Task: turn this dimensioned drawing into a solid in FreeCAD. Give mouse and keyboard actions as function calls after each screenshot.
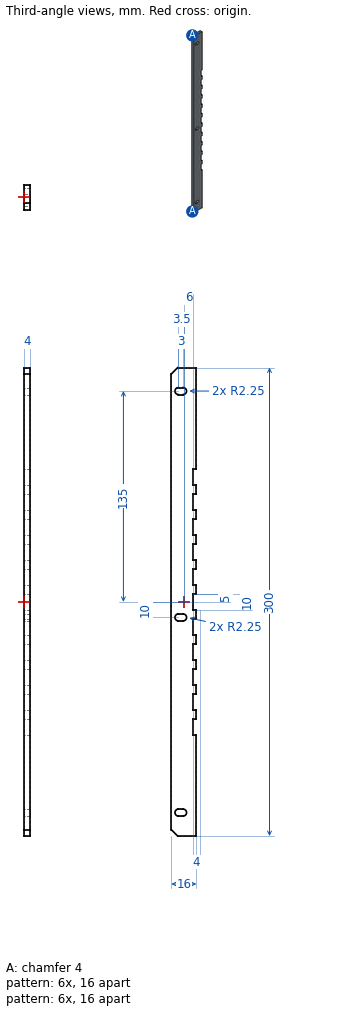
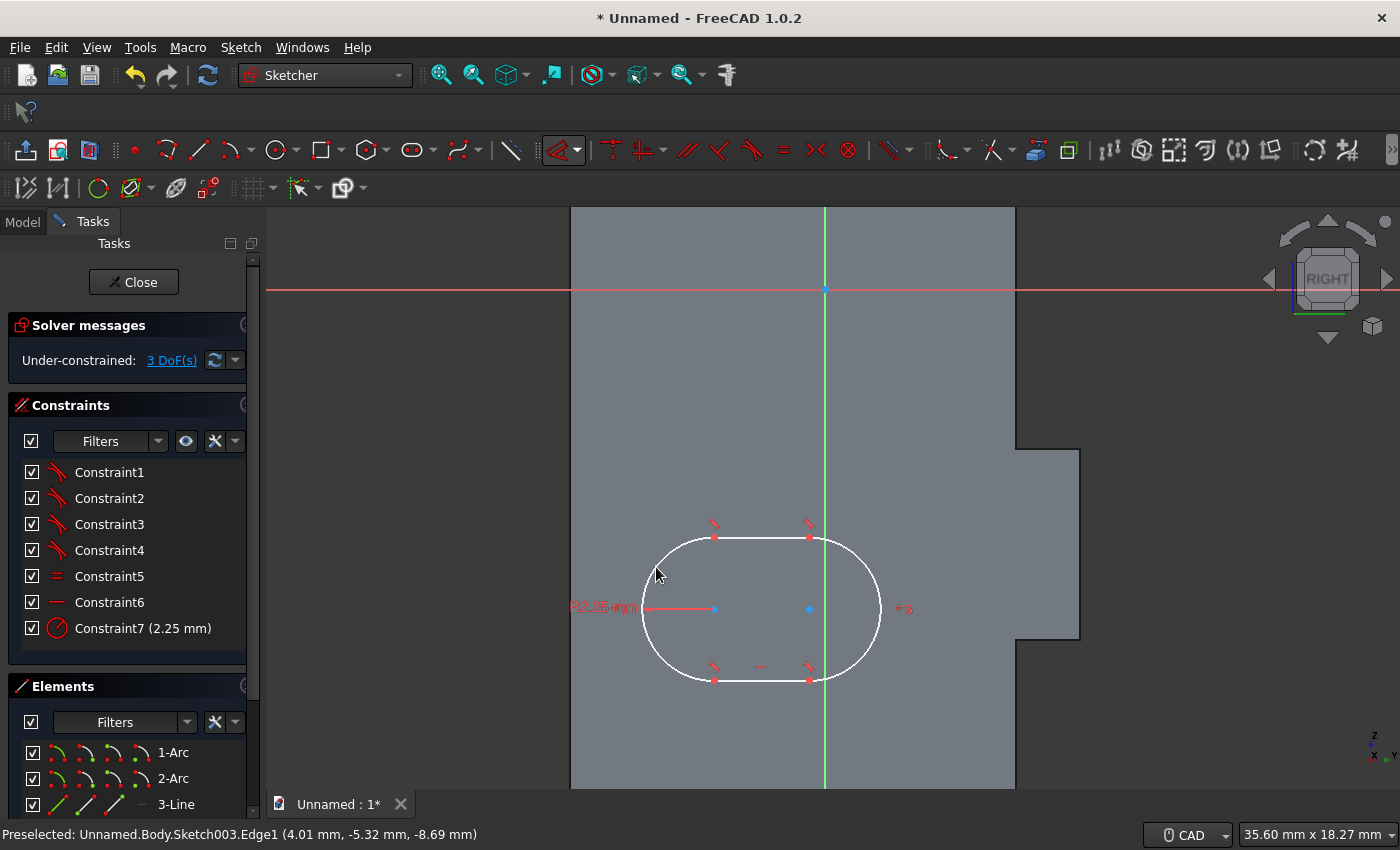
click(743, 538)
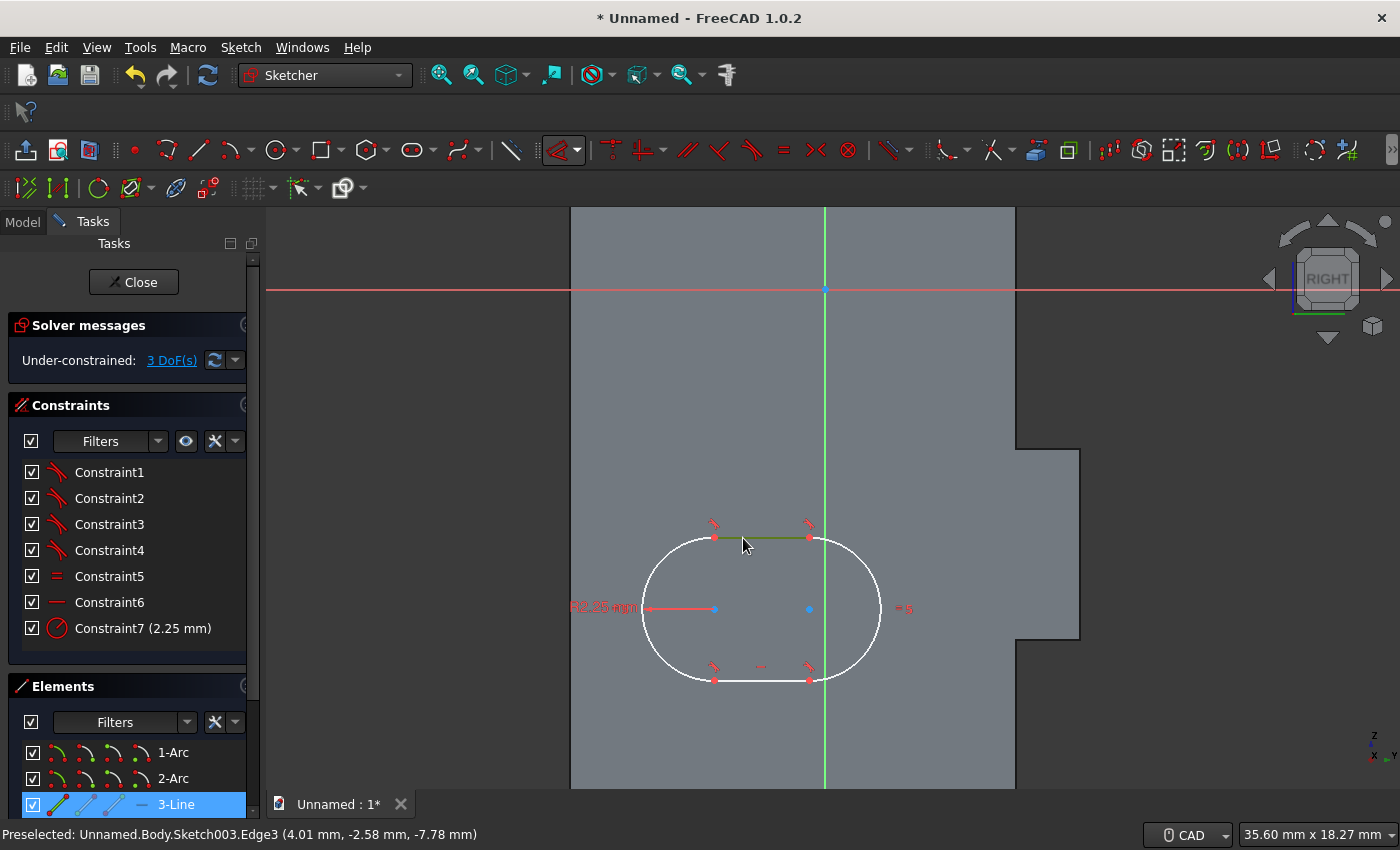
key(l)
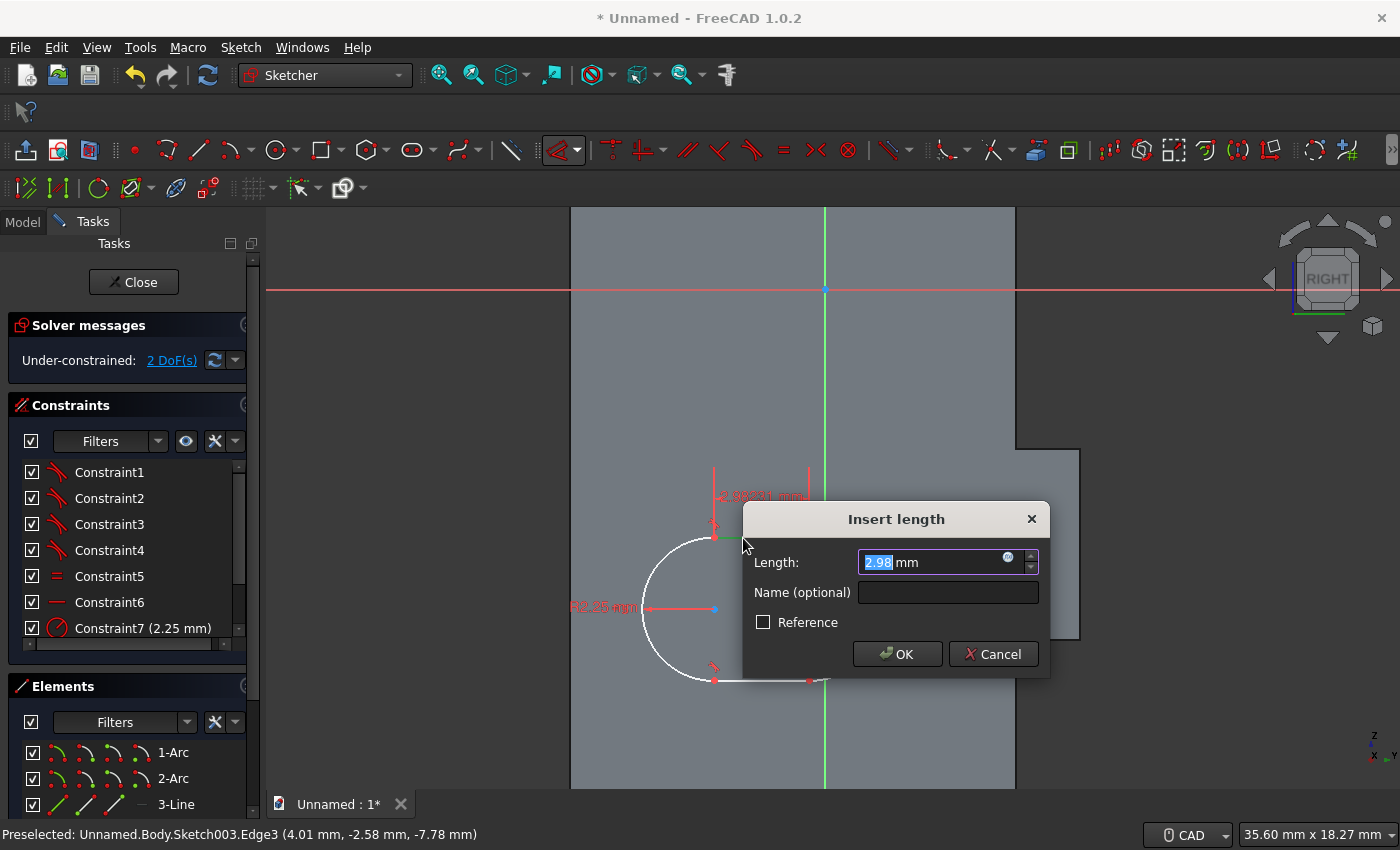
text(3)
key(Return)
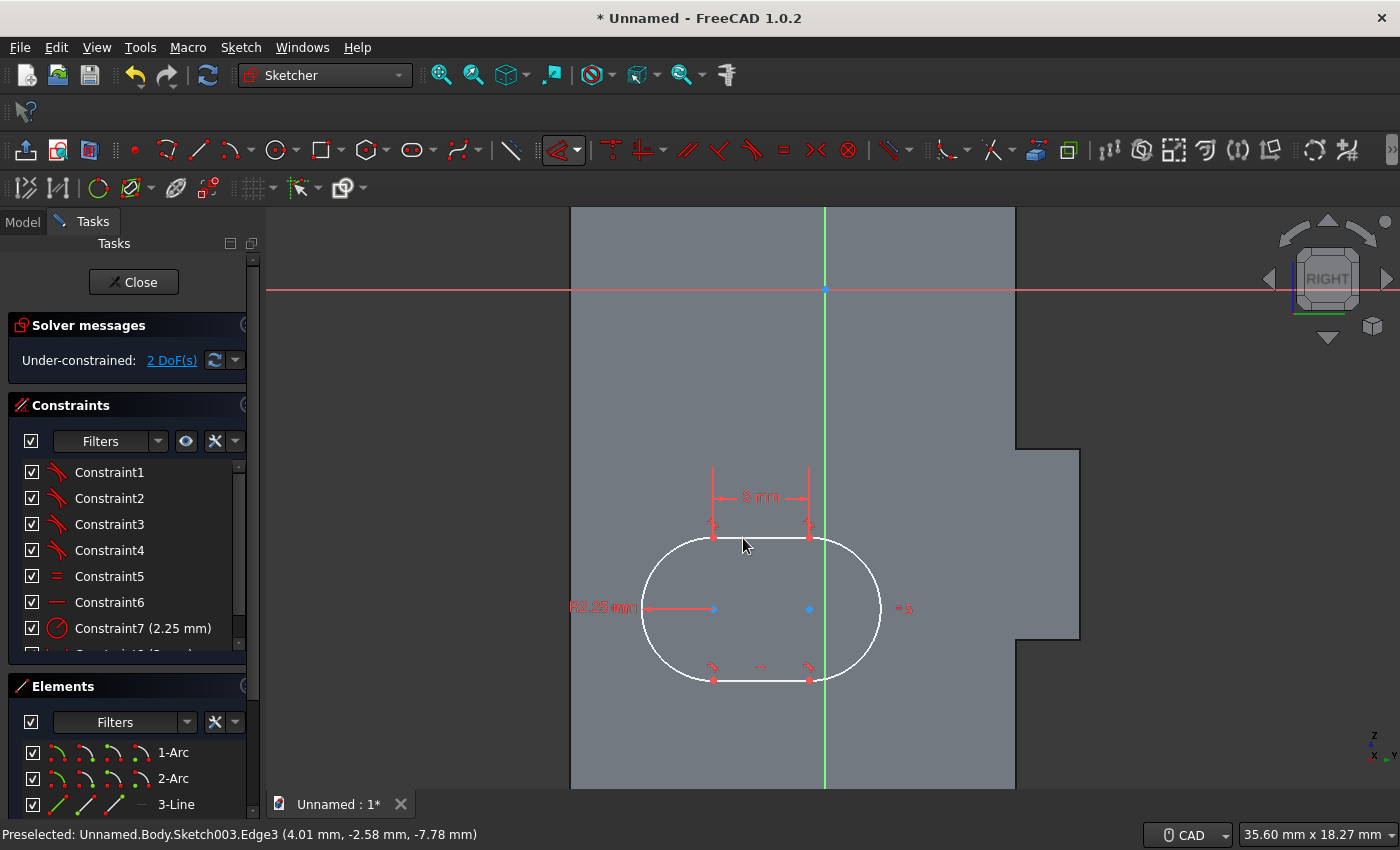
click(713, 609)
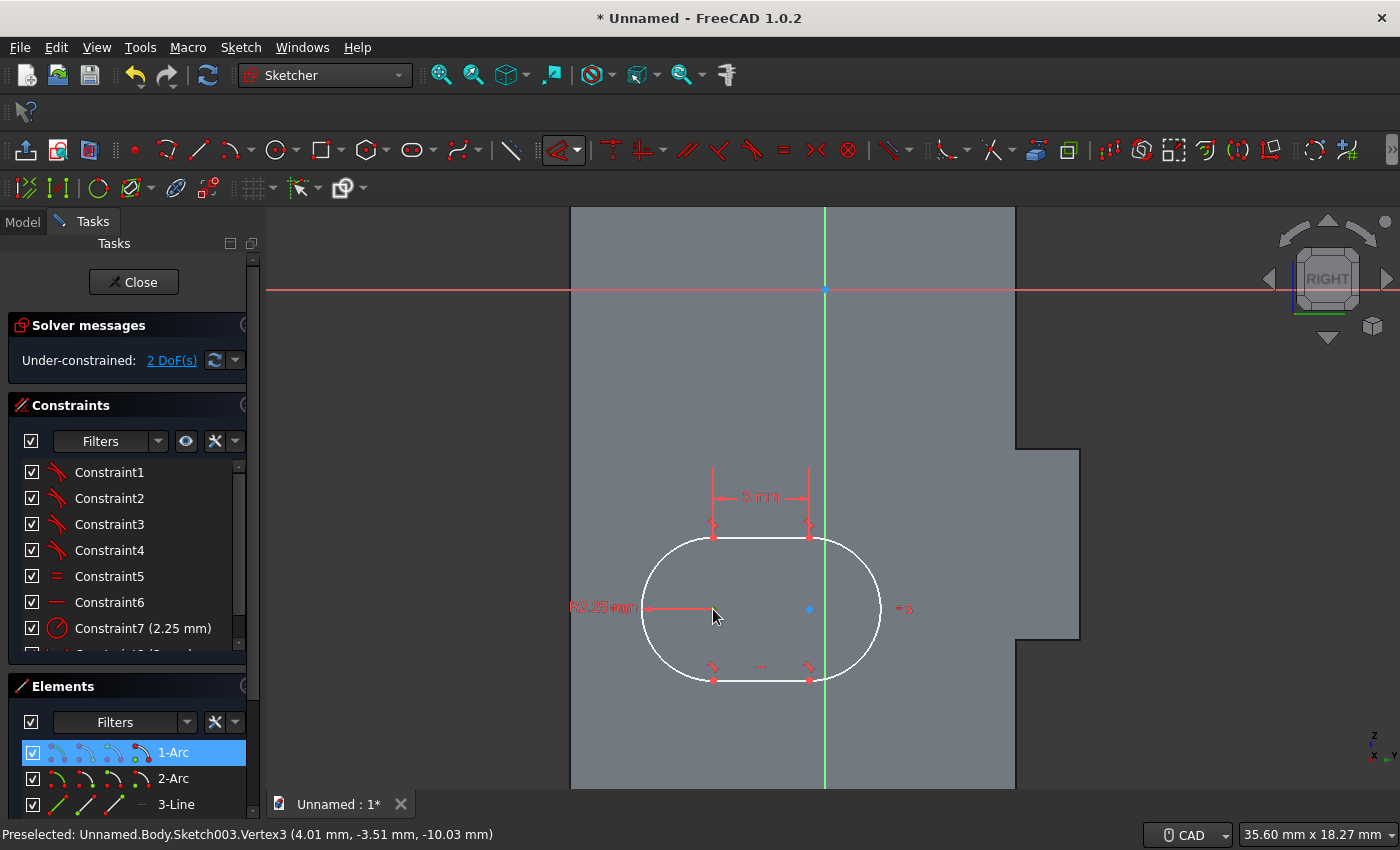
key(i)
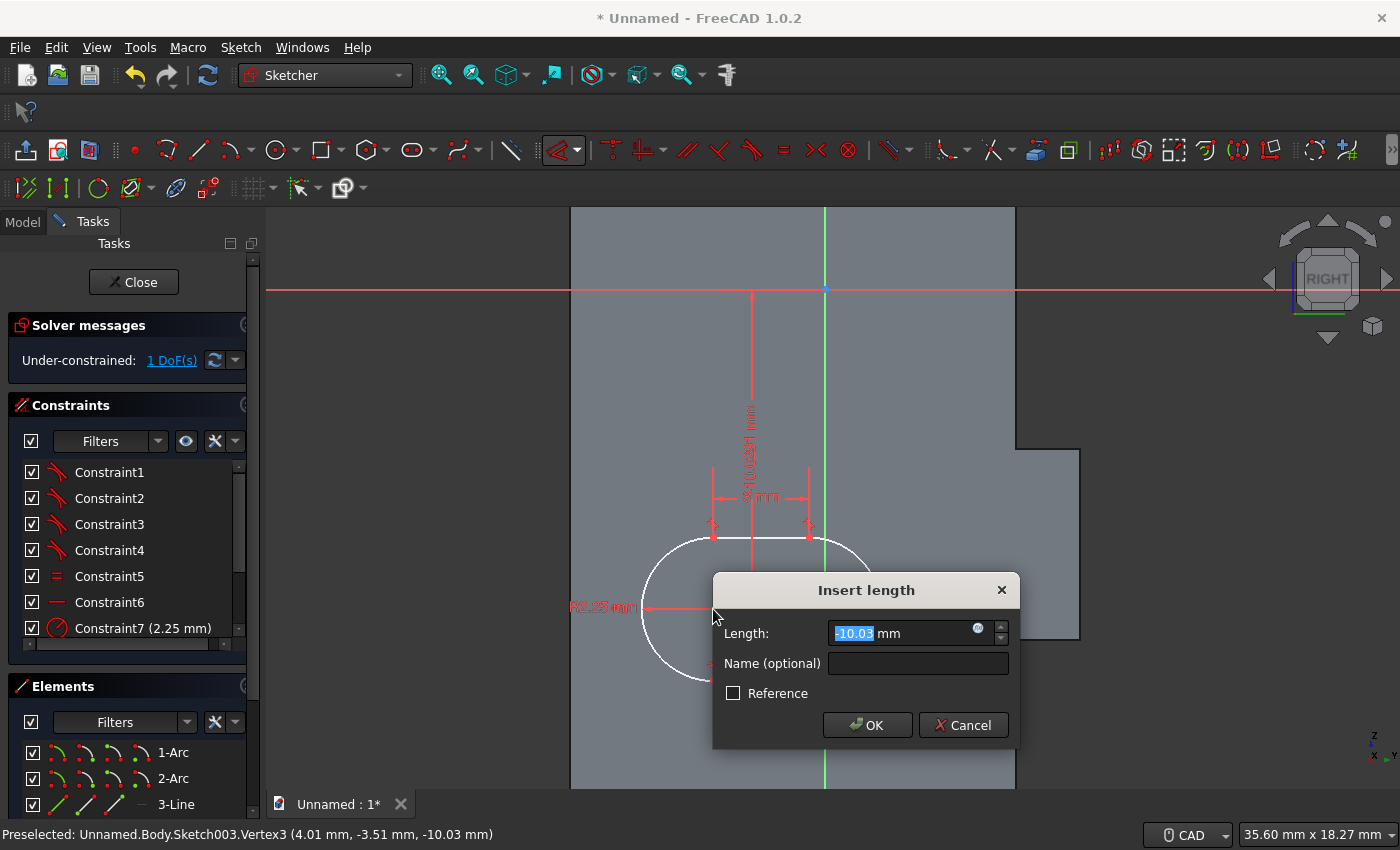
text(-10)
key(Return)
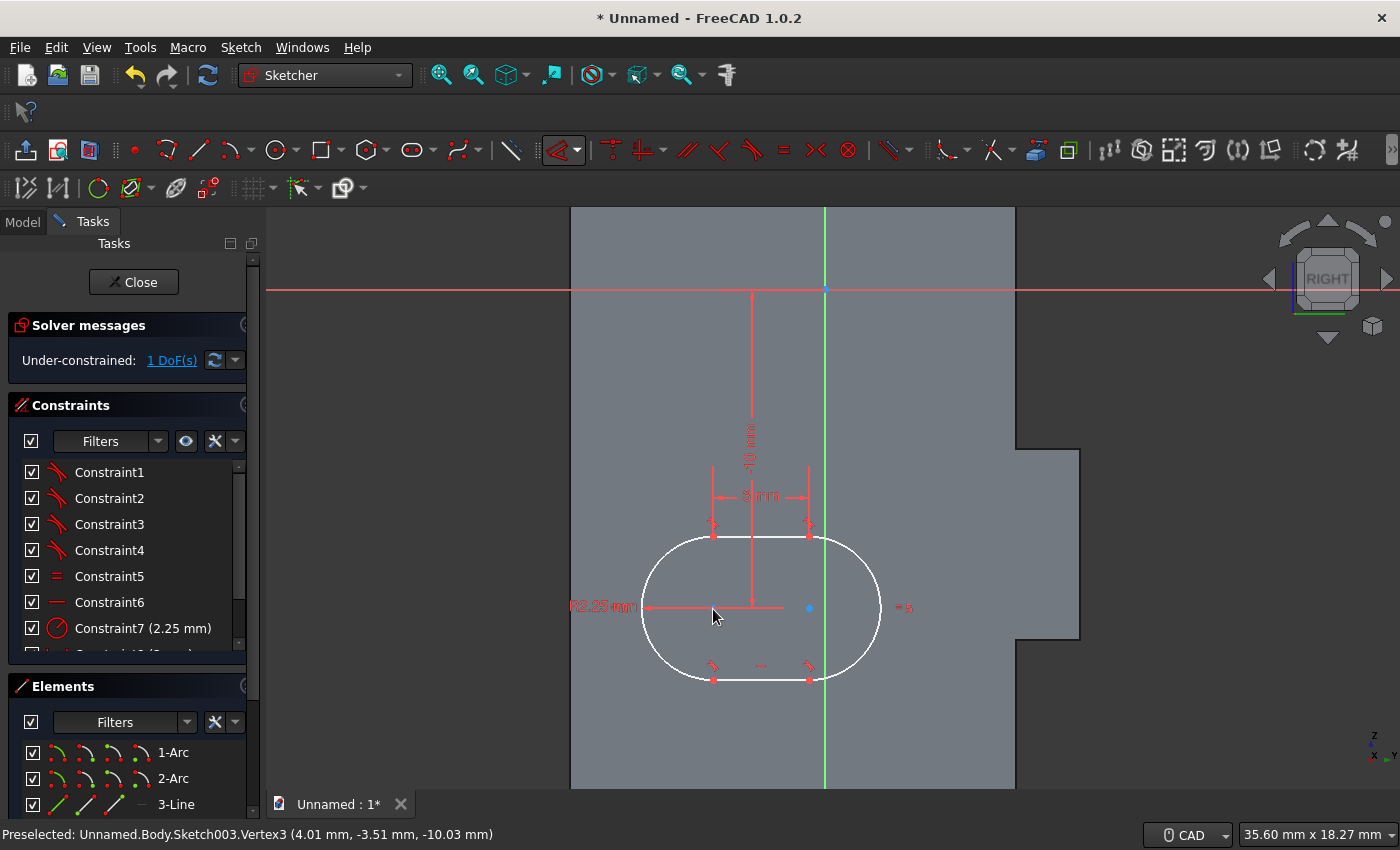
click(713, 537)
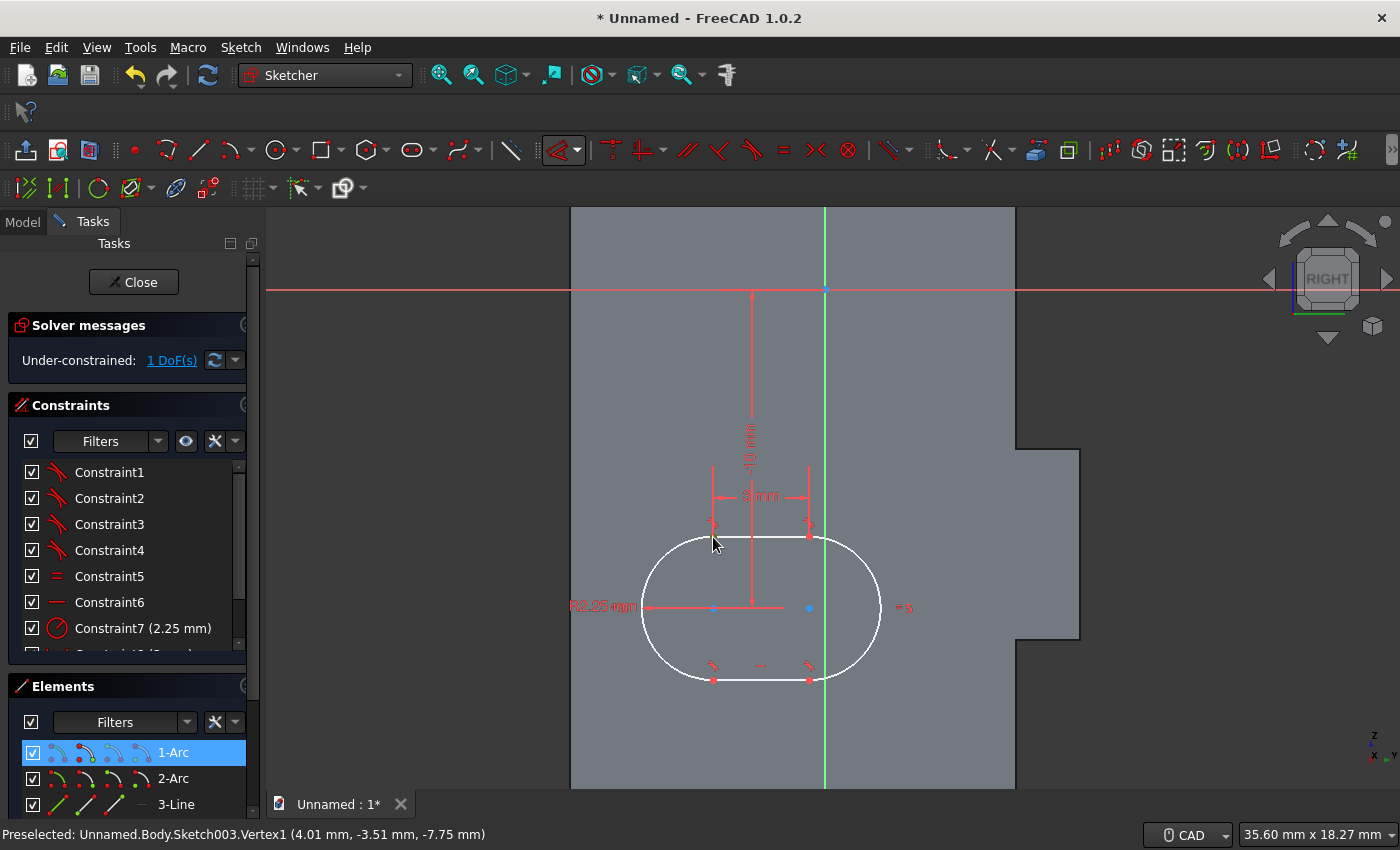
key(l)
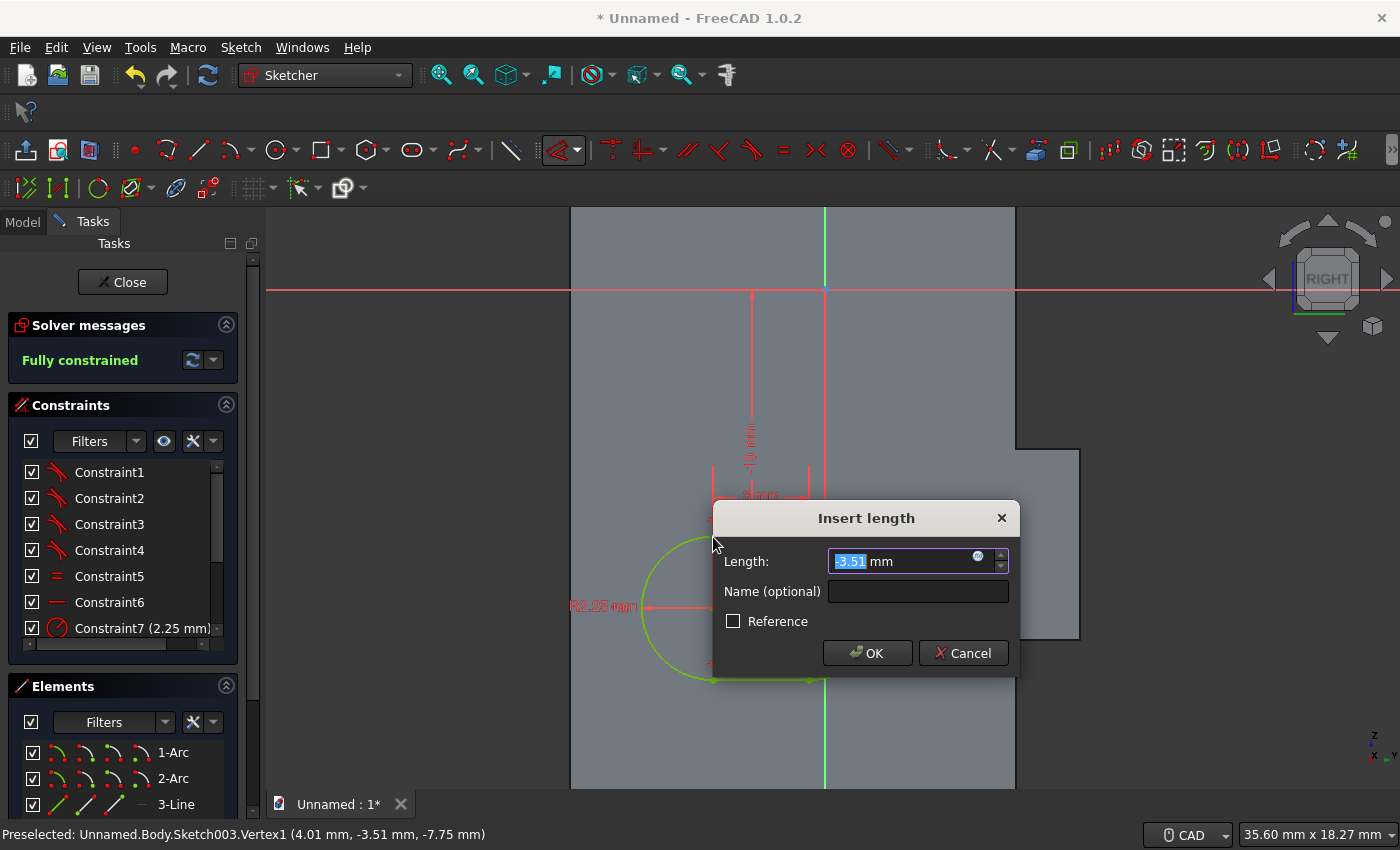
text(-3.5)
key(Return)